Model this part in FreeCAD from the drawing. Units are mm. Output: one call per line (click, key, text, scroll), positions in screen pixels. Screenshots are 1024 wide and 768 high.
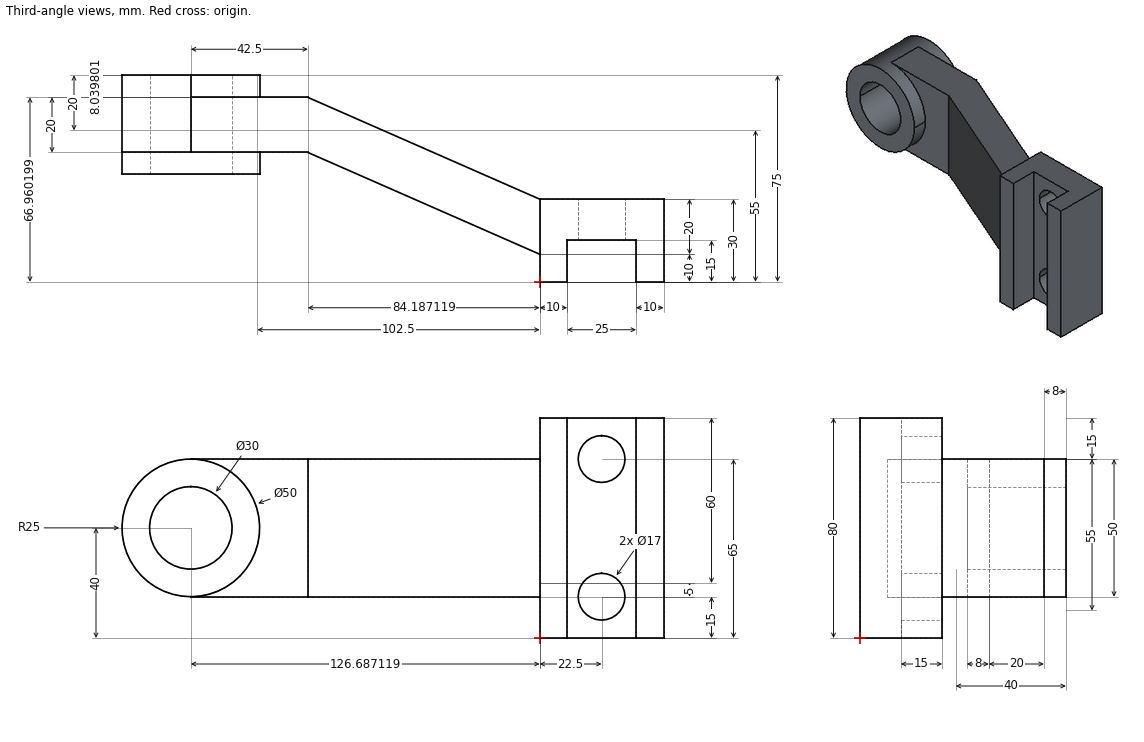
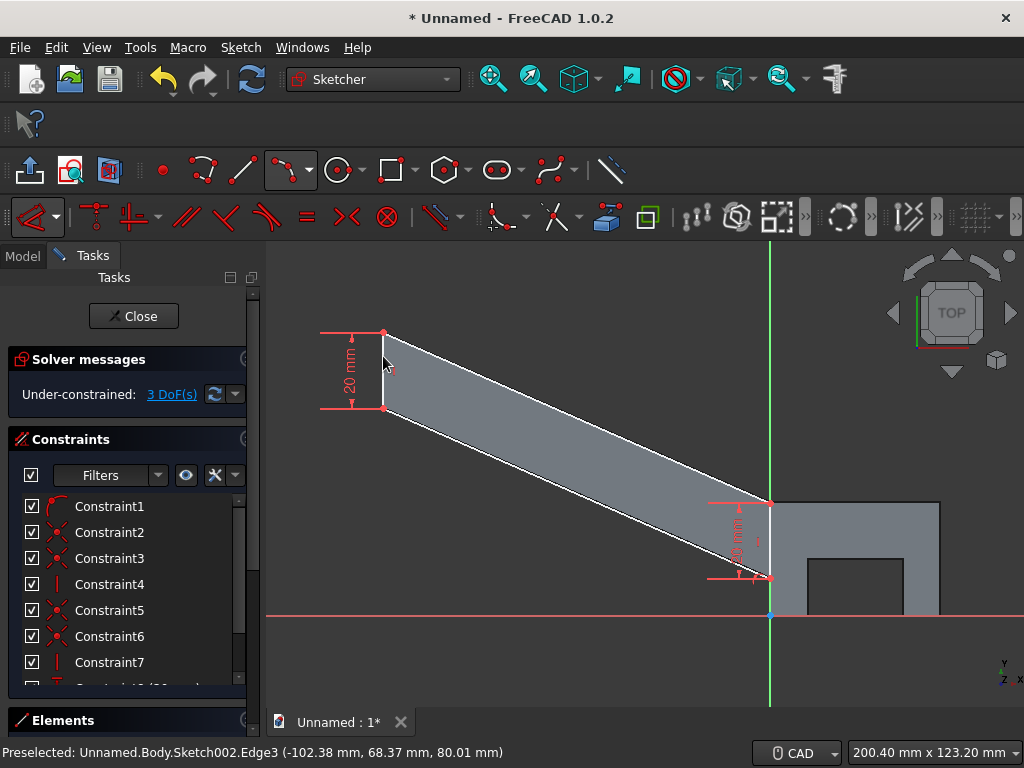
click(770, 579)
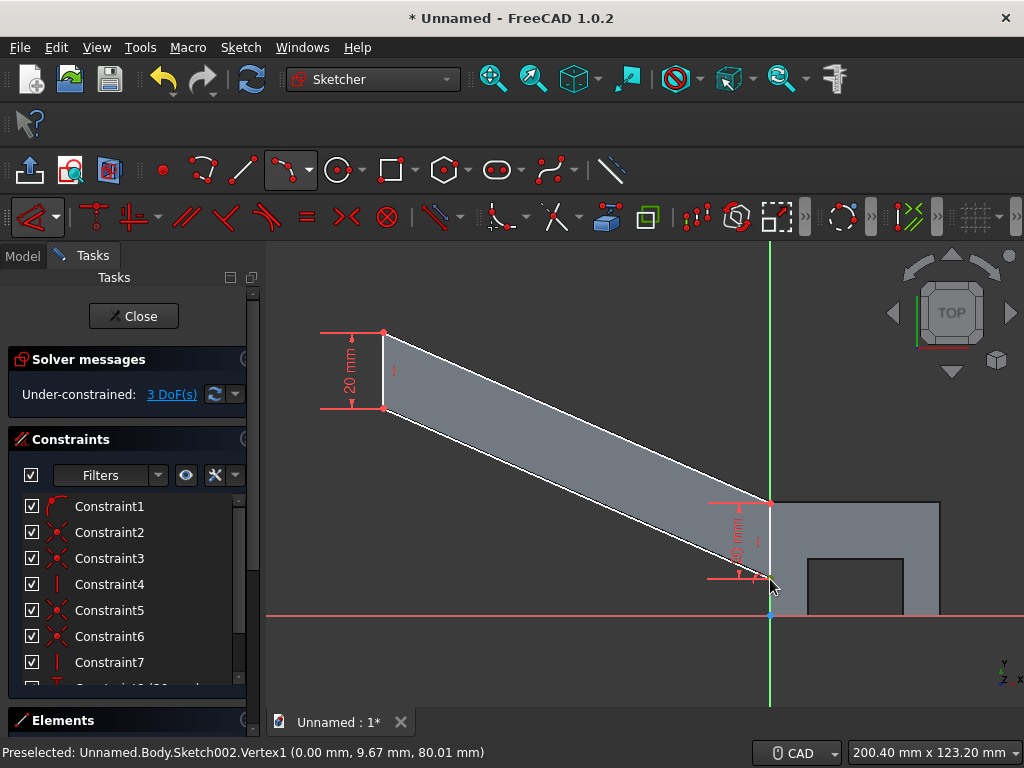
key(i)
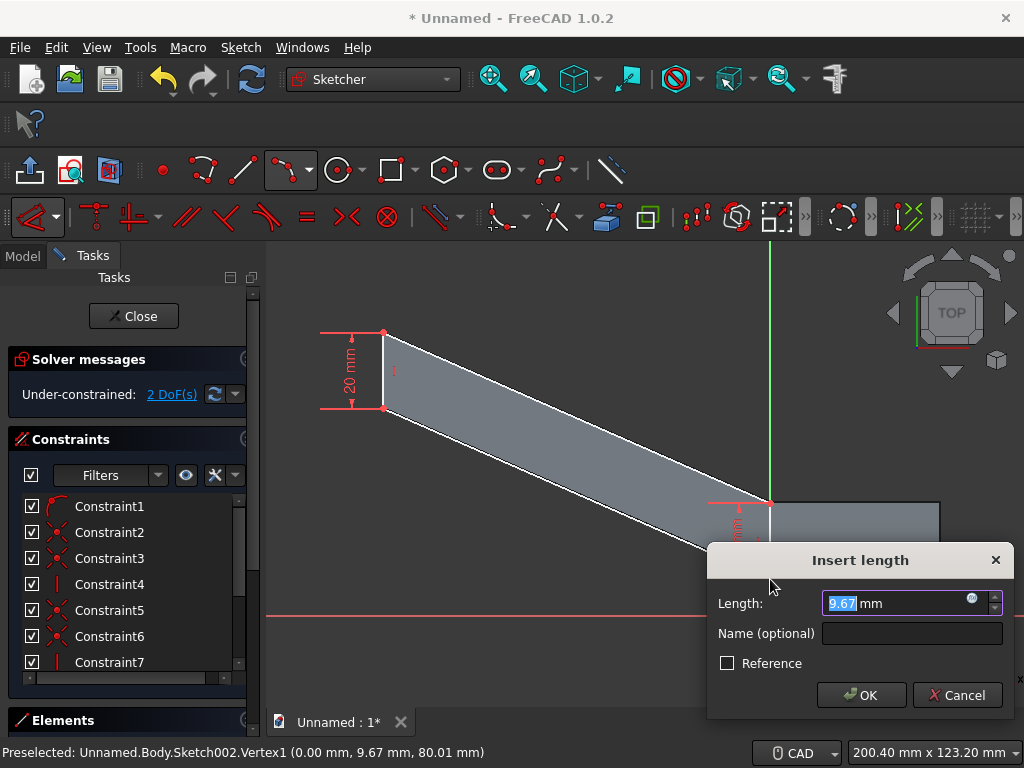
text(10)
key(Return)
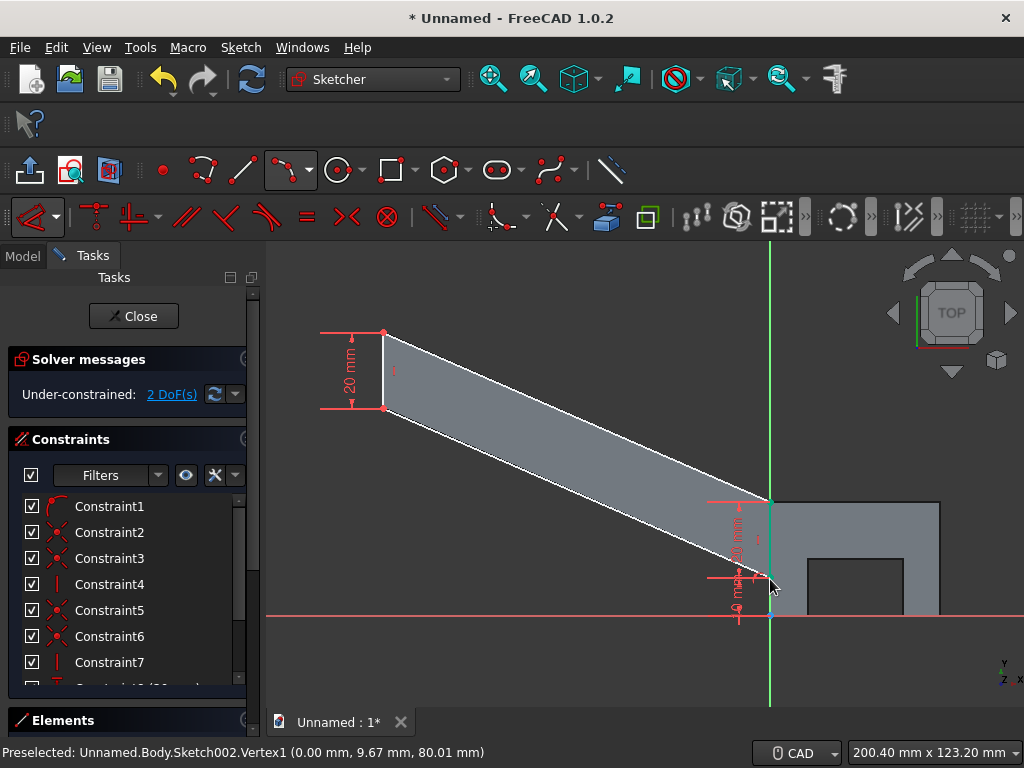
click(383, 333)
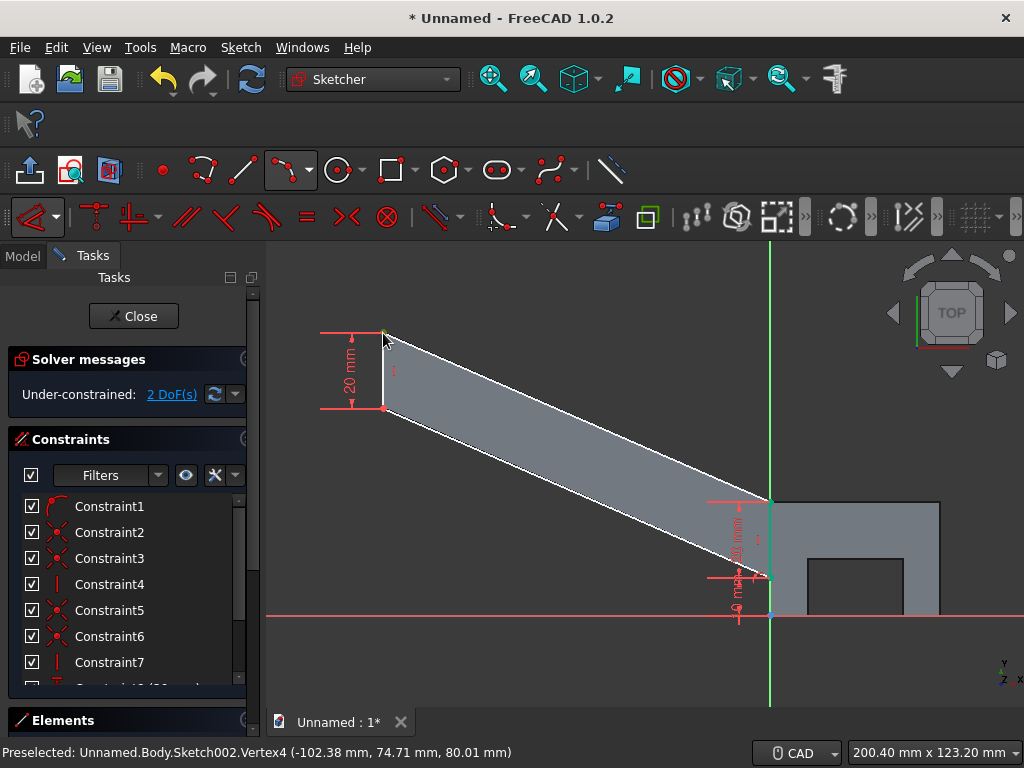
key(i)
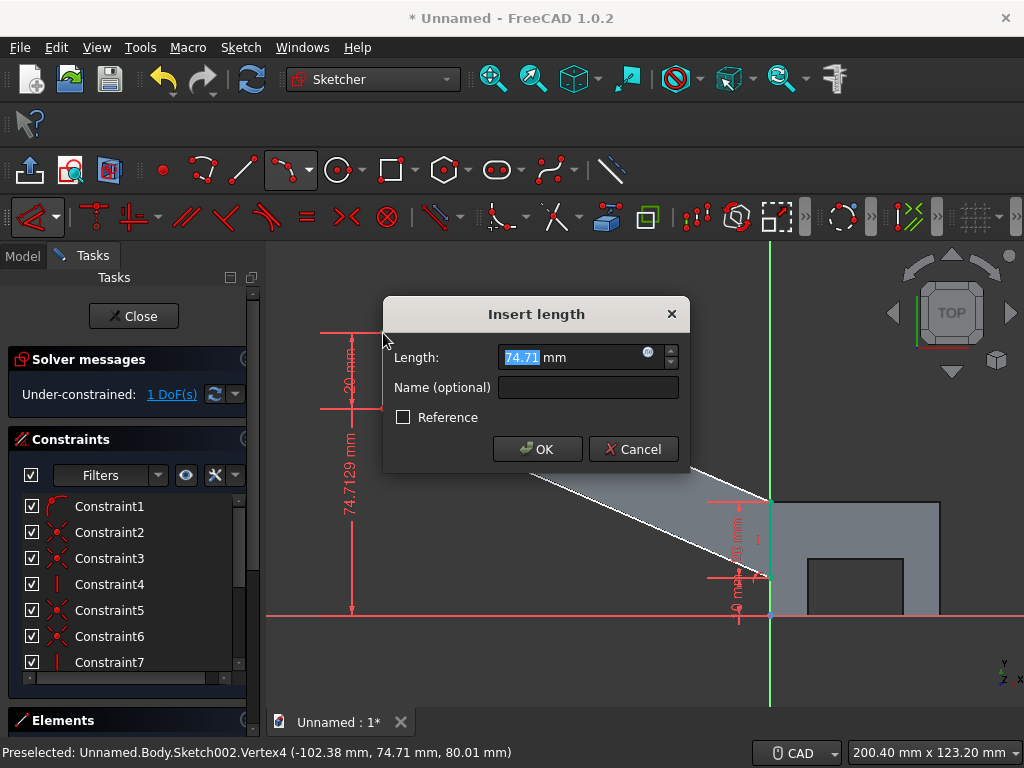
text(75)
key(Return)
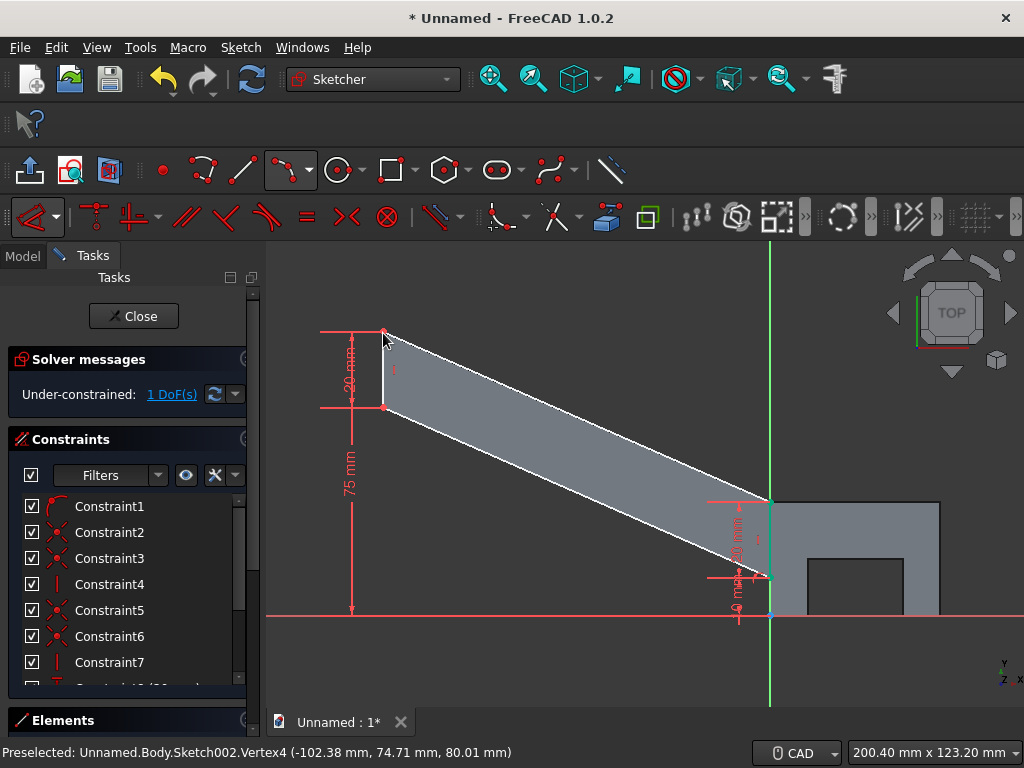
click(383, 332)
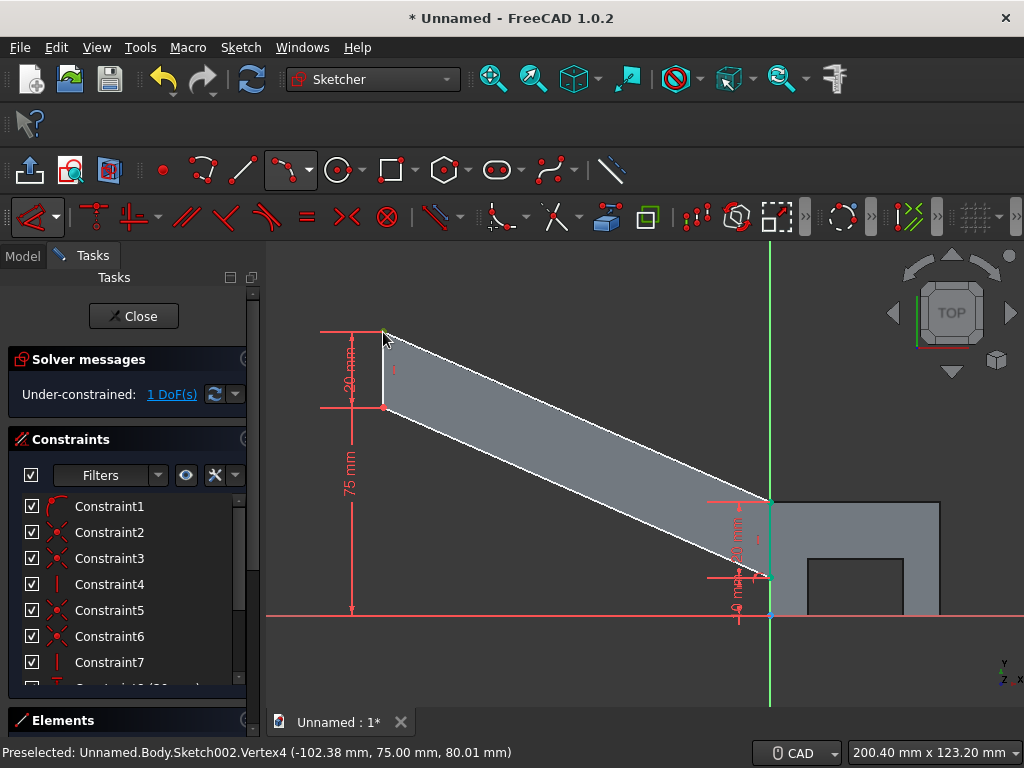
key(l)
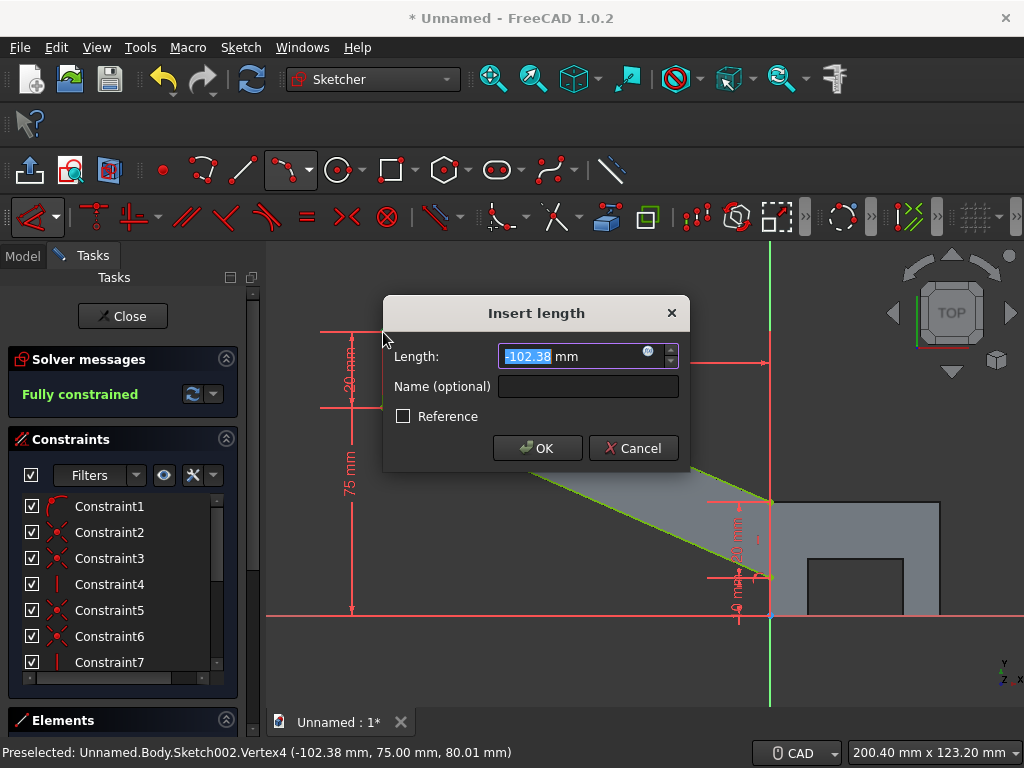
text(-102.5)
key(Return)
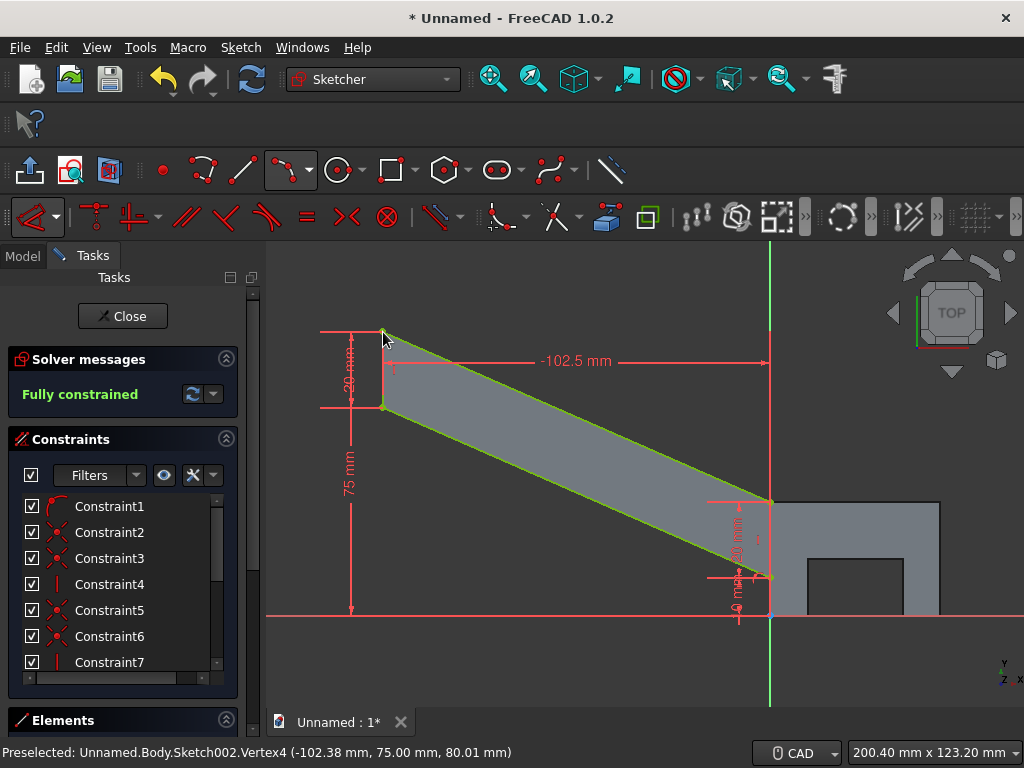
click(123, 316)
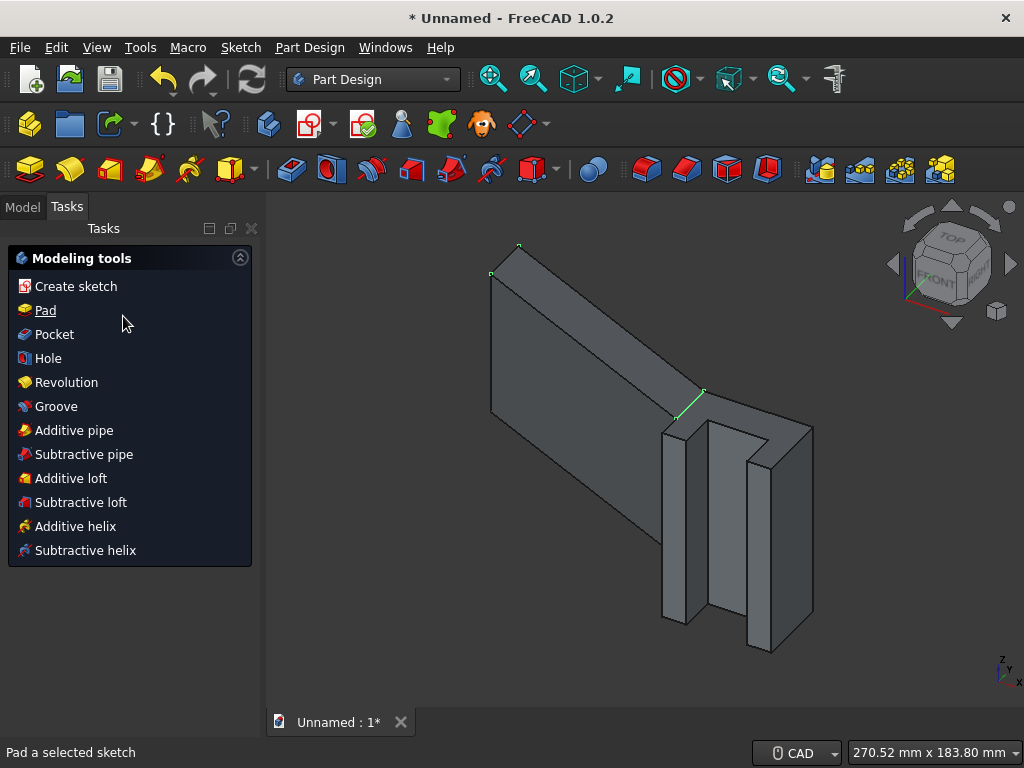
click(292, 170)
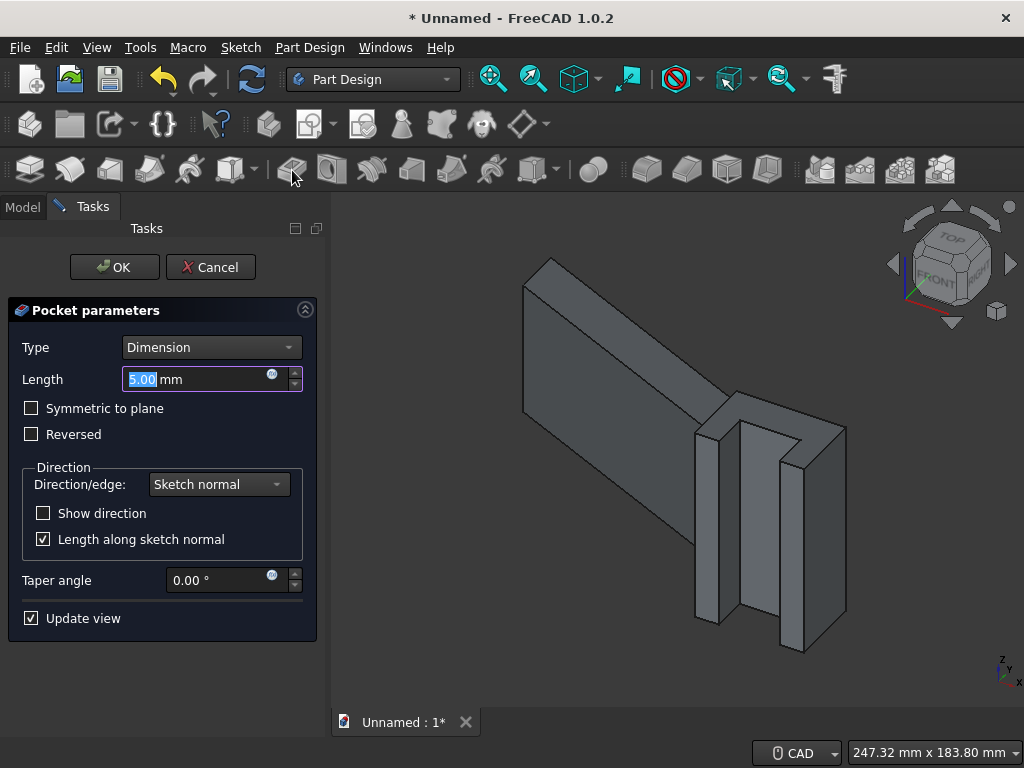
text(15)
key(Tab)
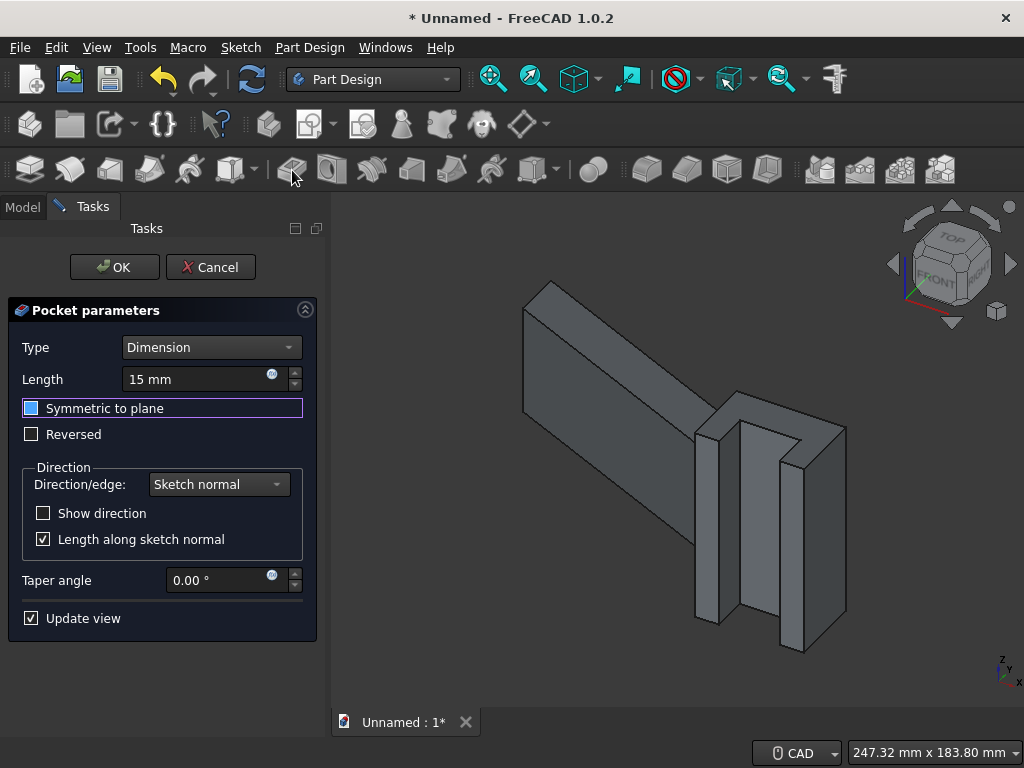
click(115, 267)